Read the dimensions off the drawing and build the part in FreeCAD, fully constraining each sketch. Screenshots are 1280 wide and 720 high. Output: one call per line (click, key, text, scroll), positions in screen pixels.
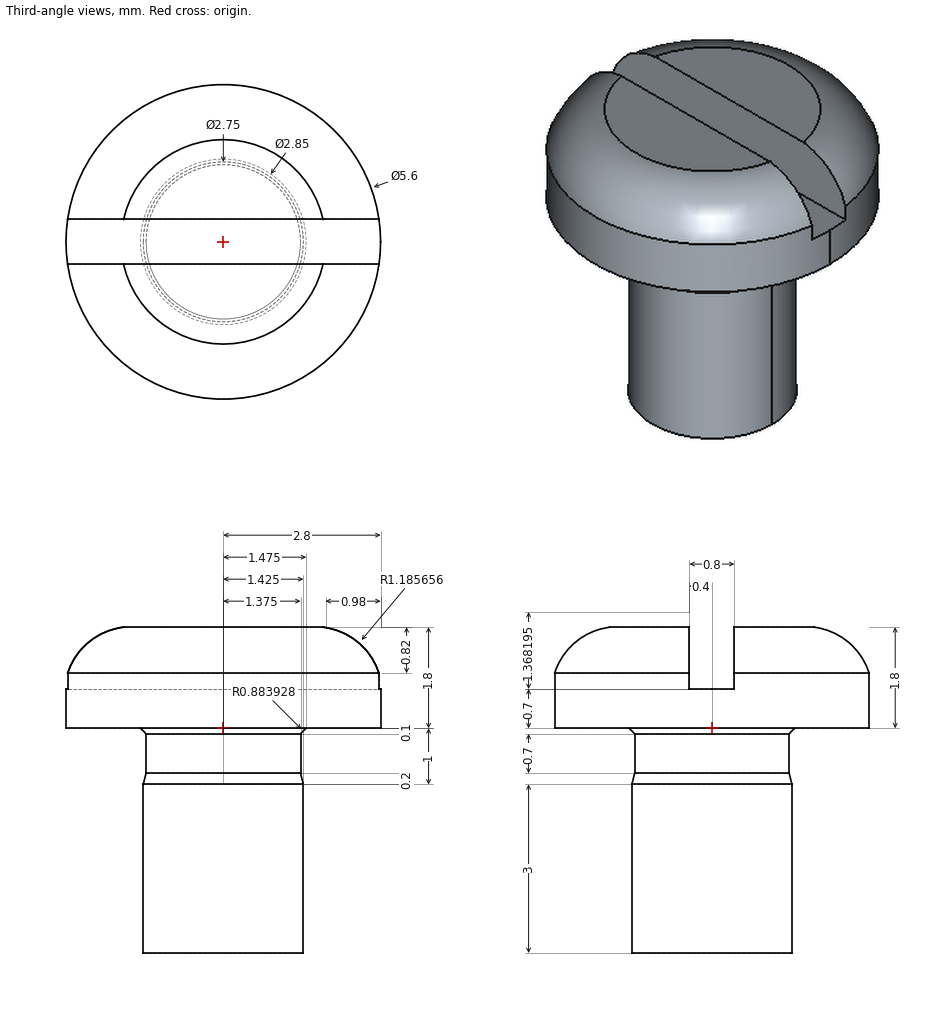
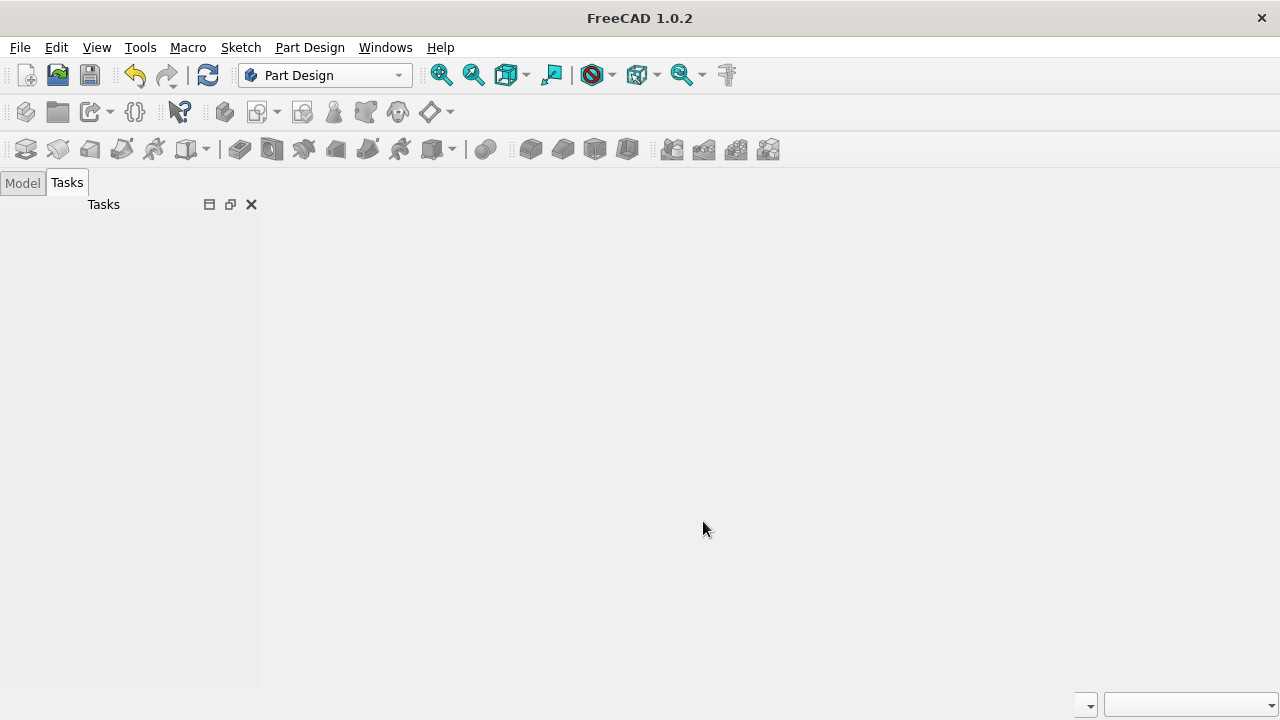
click(26, 76)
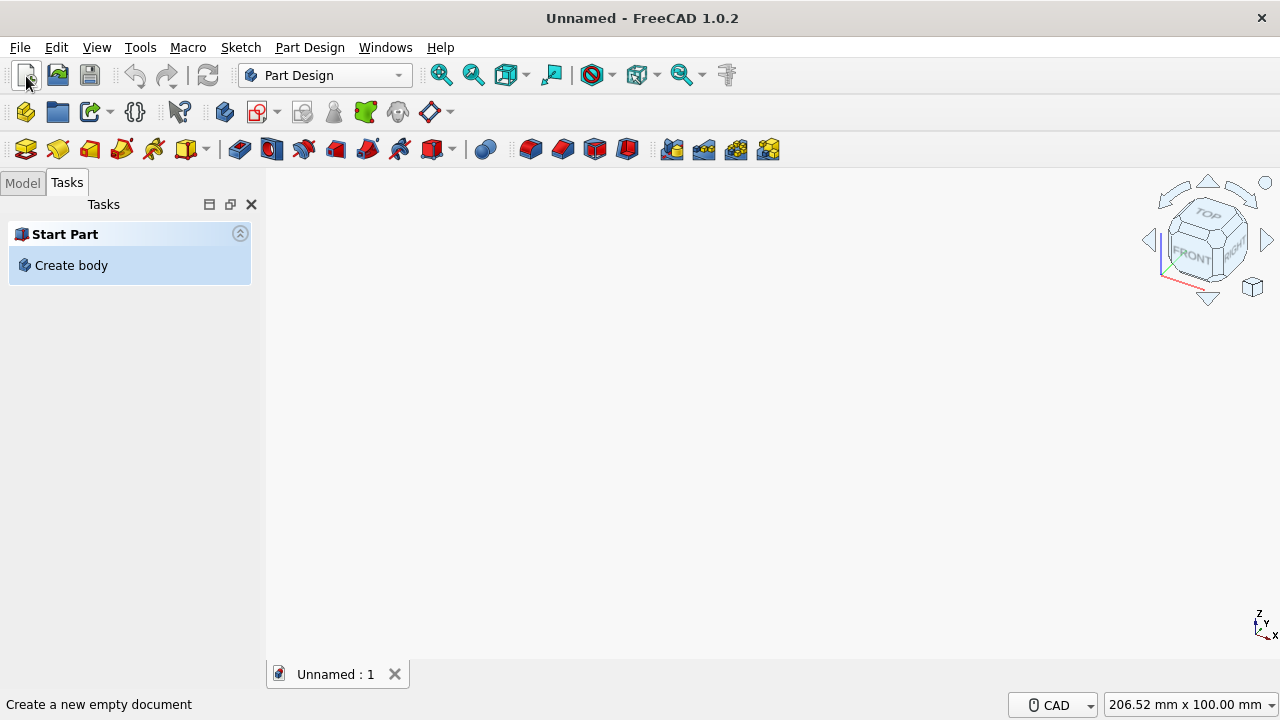
click(258, 112)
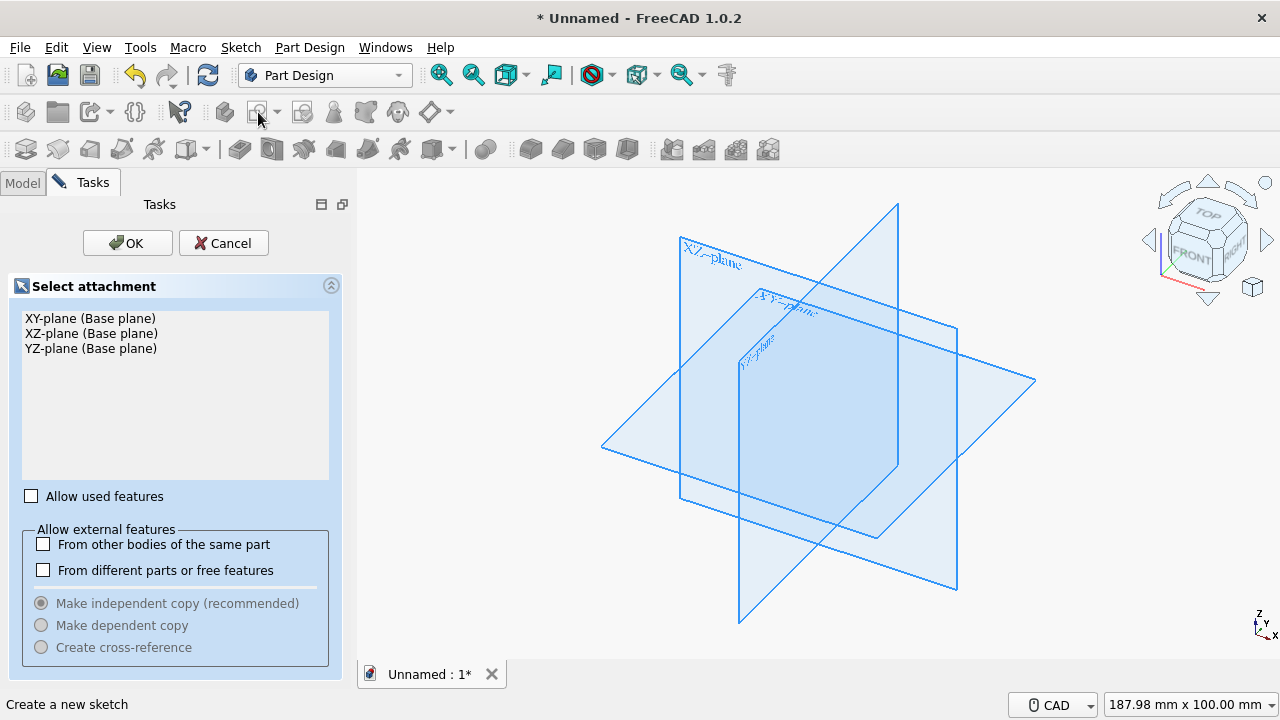
click(82, 318)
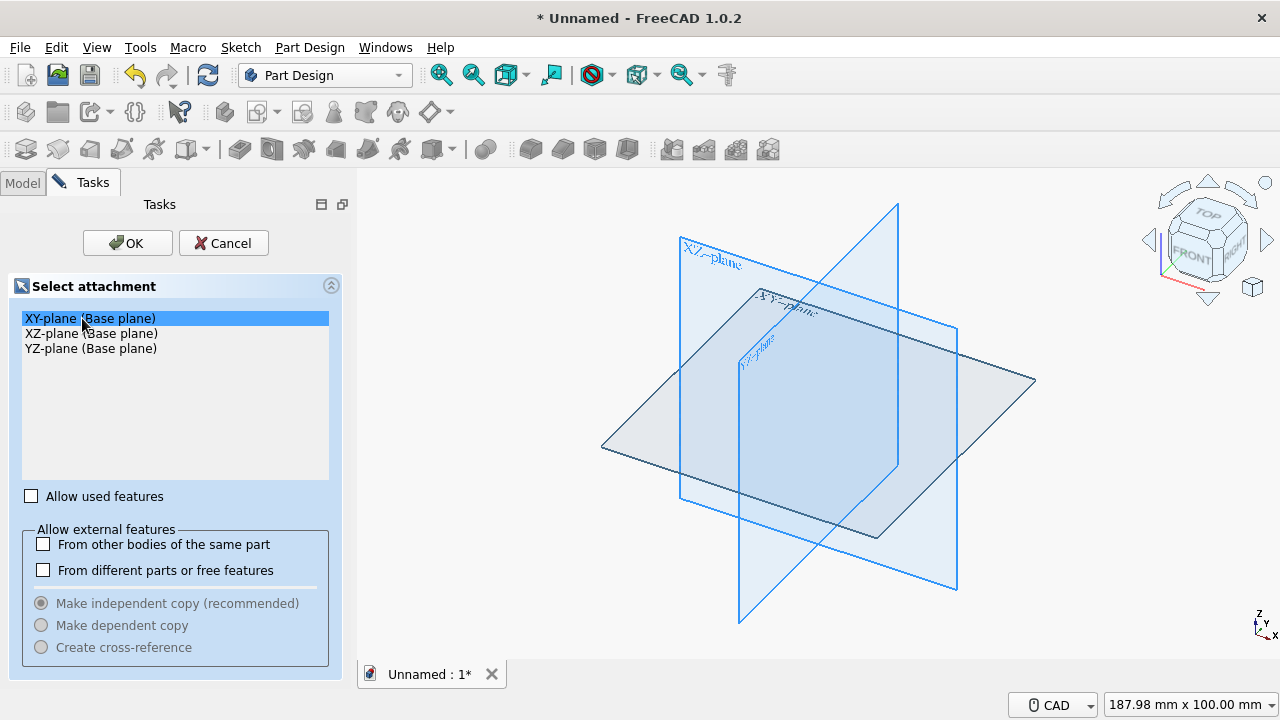
click(128, 243)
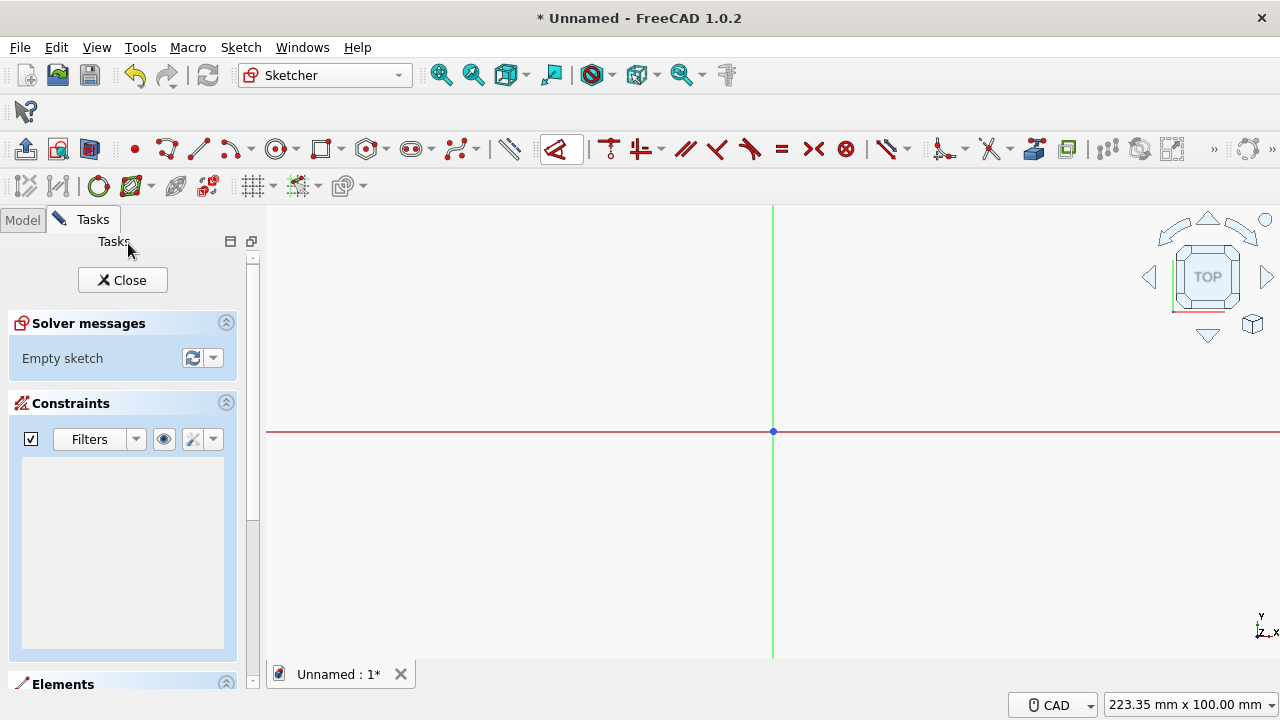
scroll(780, 432, up, 12)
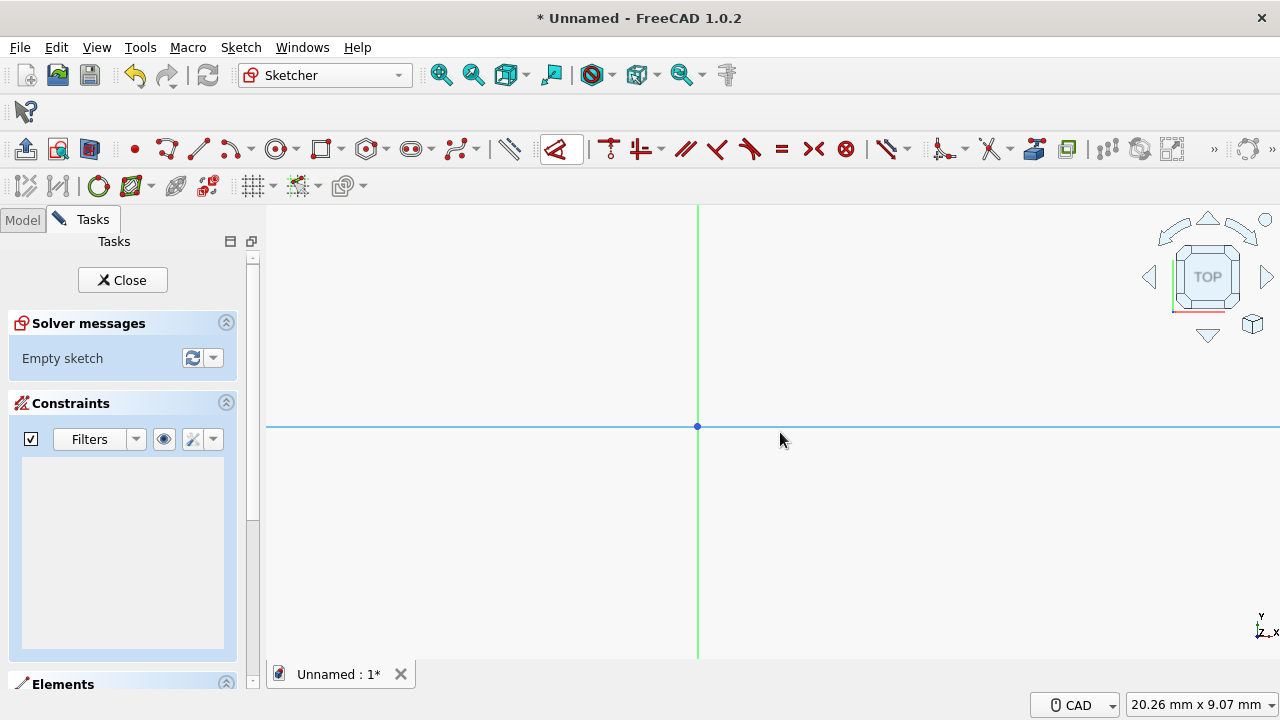
click(276, 150)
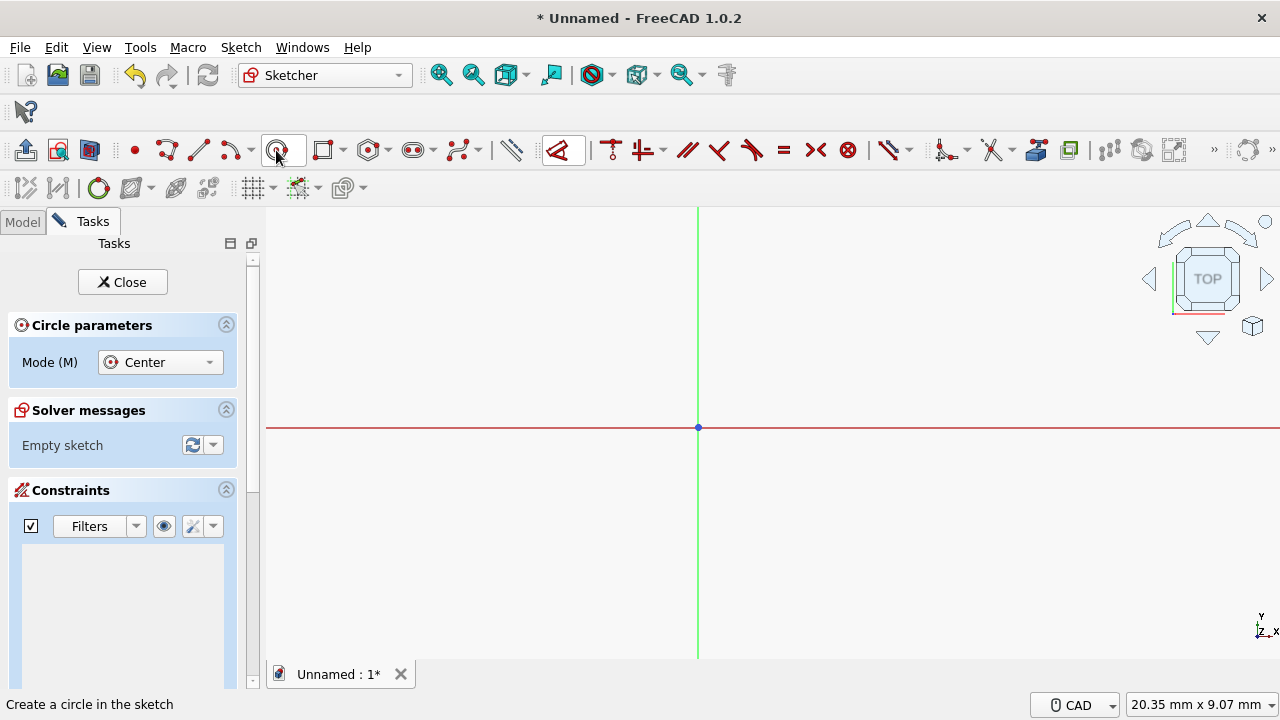
click(698, 428)
click(797, 329)
key(Escape)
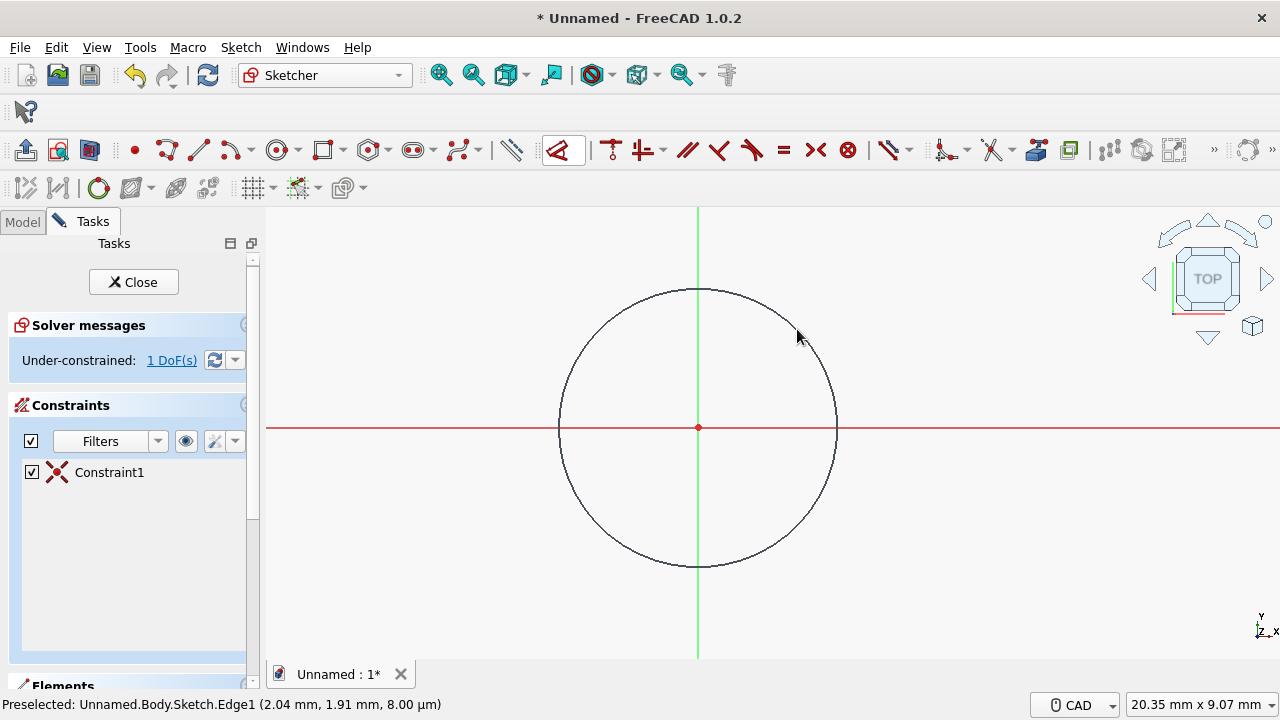
click(796, 329)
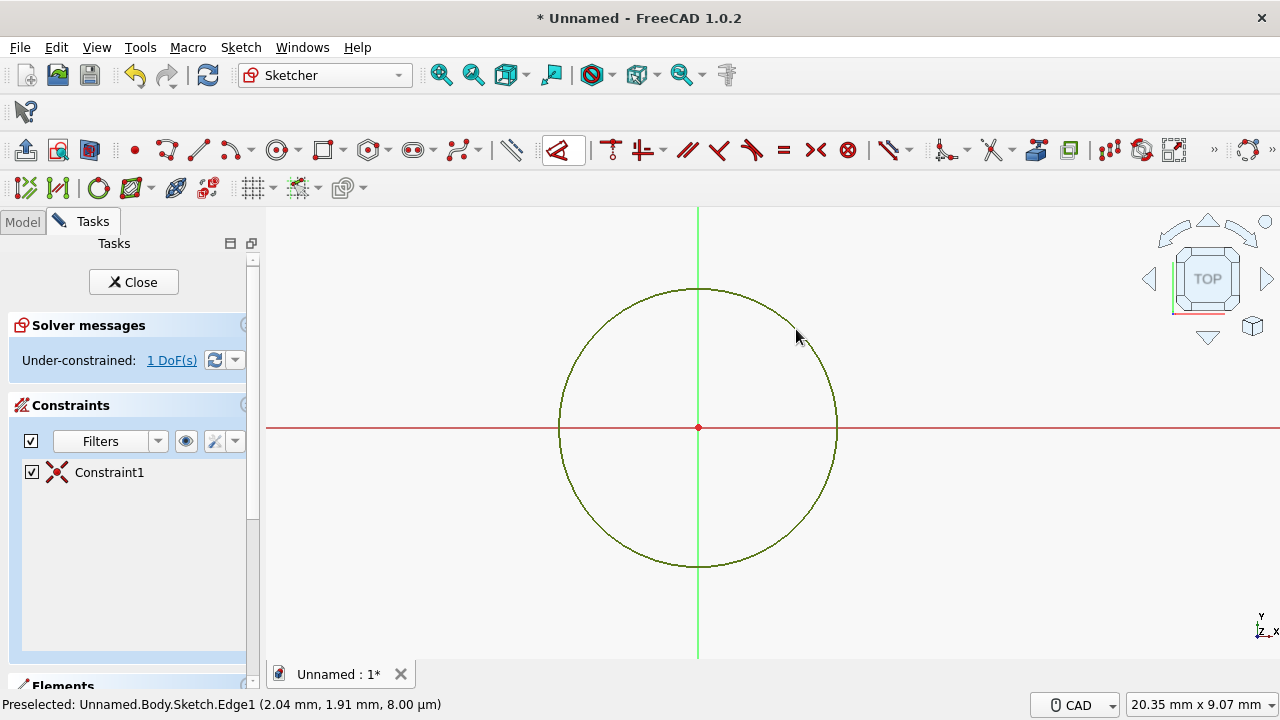
click(580, 150)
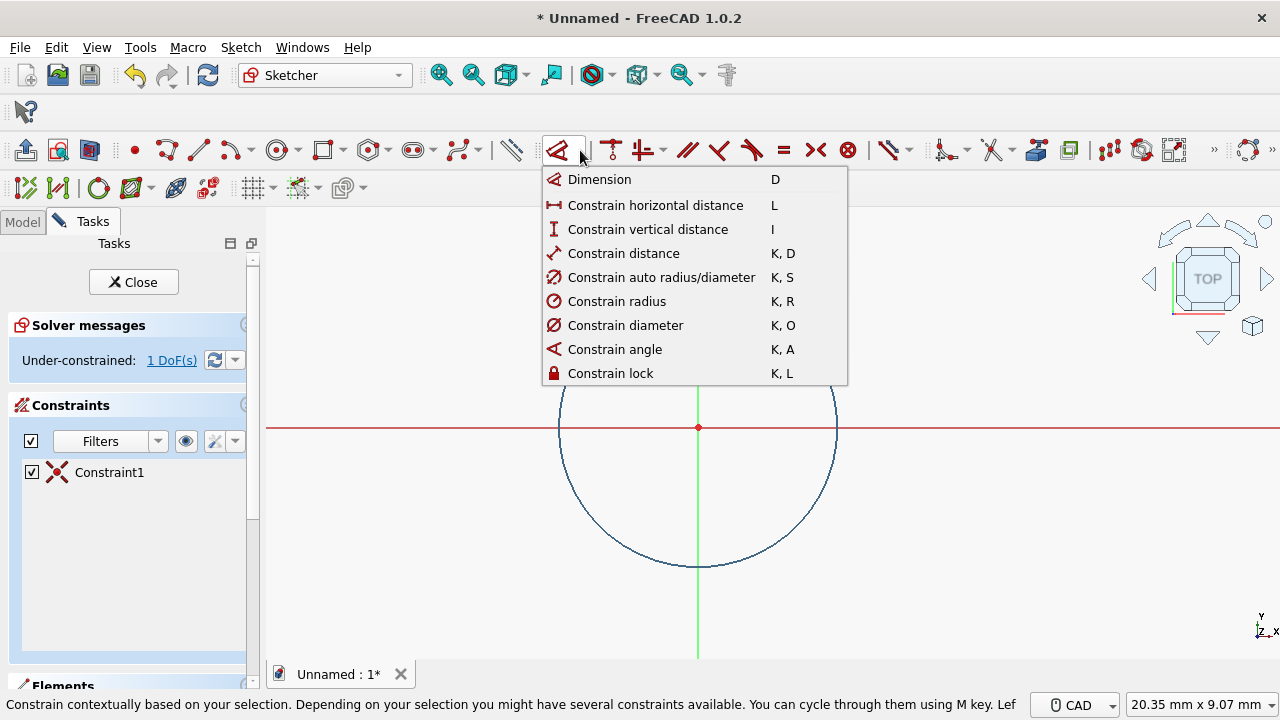
click(695, 325)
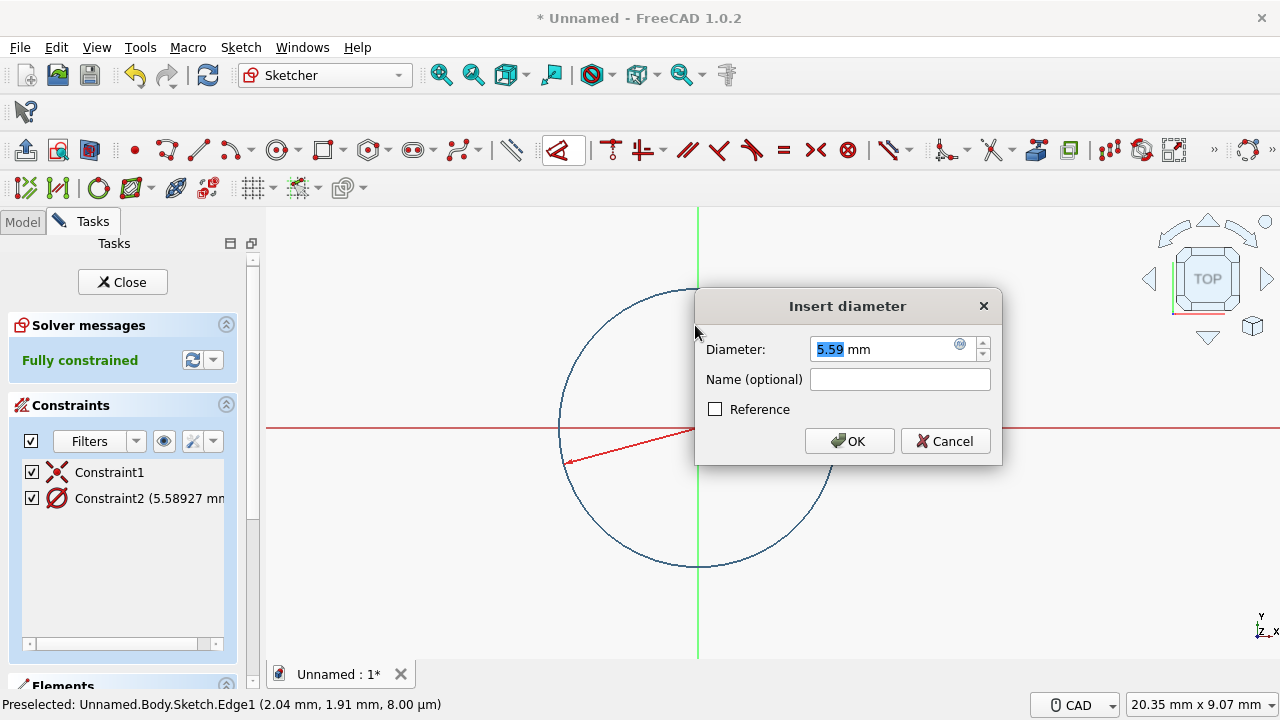
text(5.6)
key(Return)